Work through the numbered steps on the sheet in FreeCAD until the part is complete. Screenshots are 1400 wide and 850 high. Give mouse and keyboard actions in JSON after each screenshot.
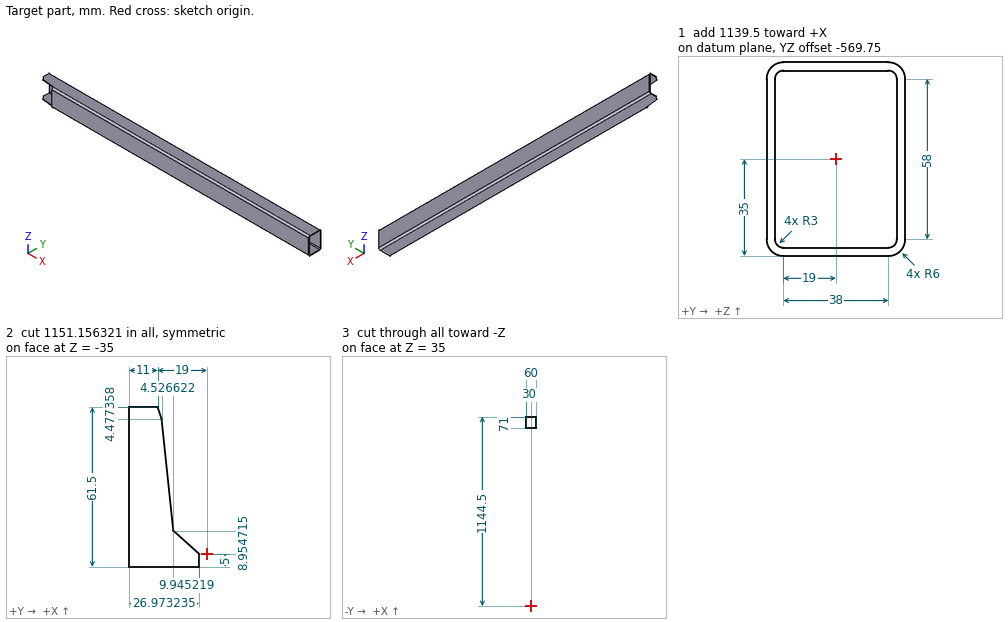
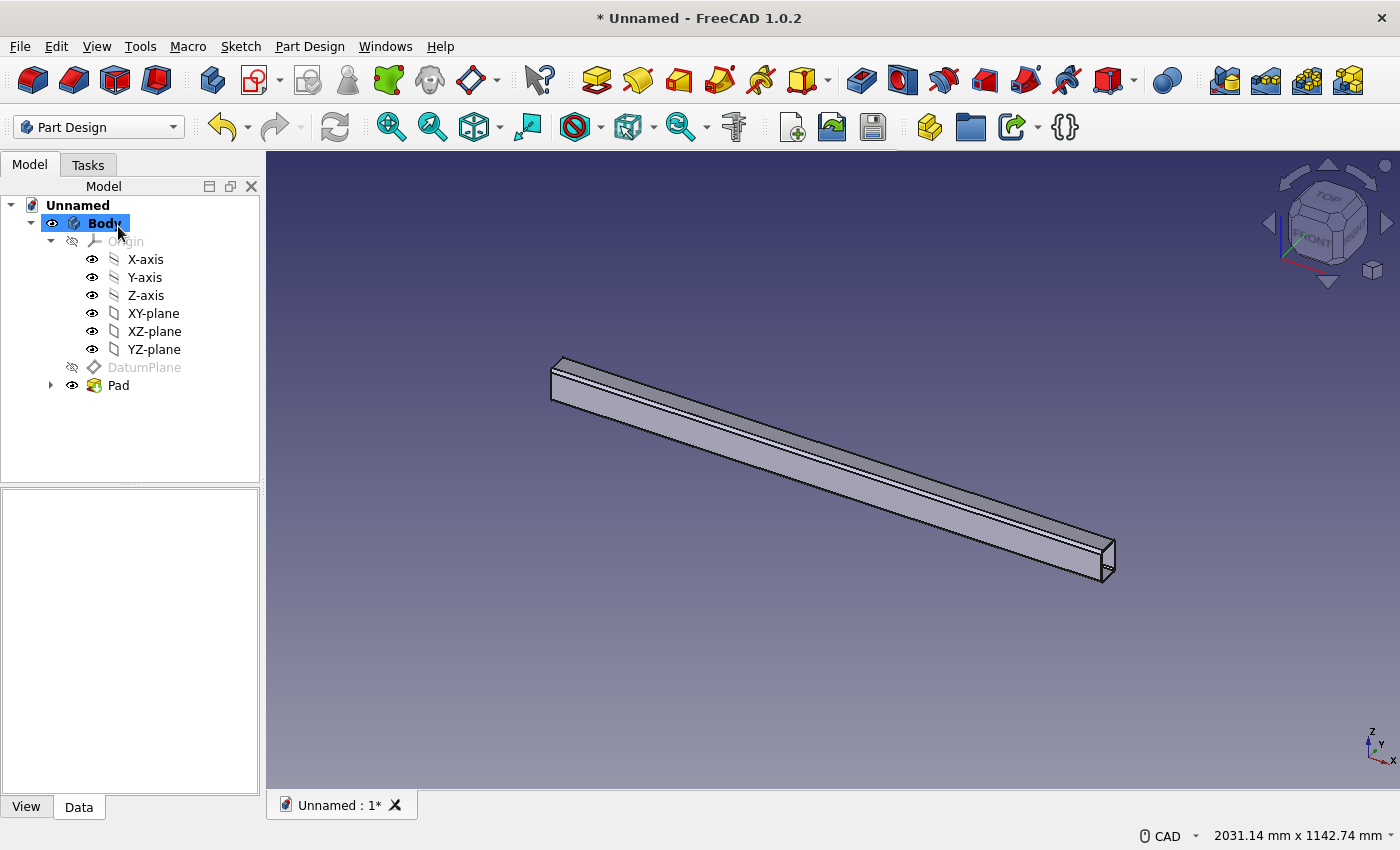
{"action": "key", "text": "5"}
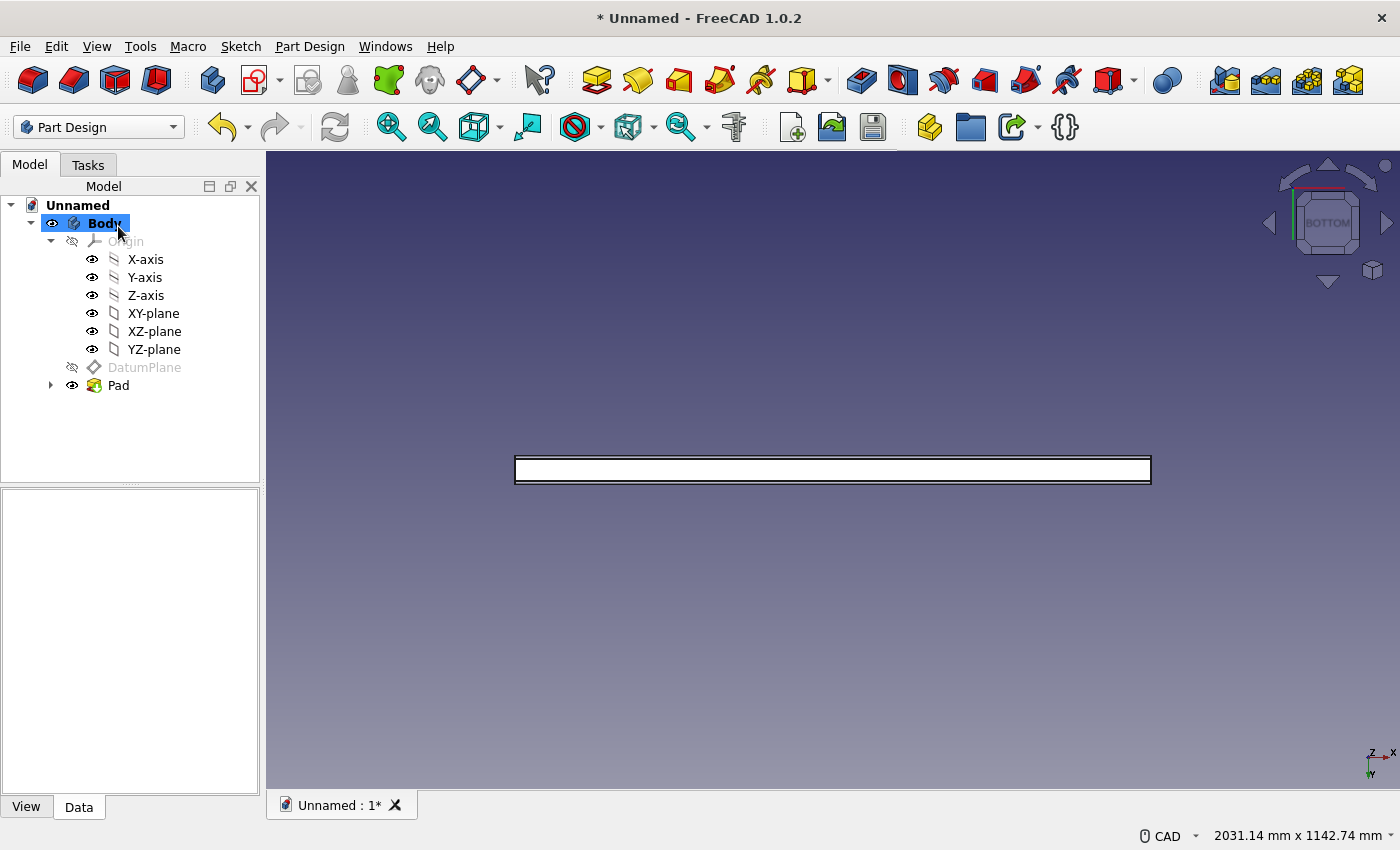
{"action": "left_click", "coordinate": [833, 469]}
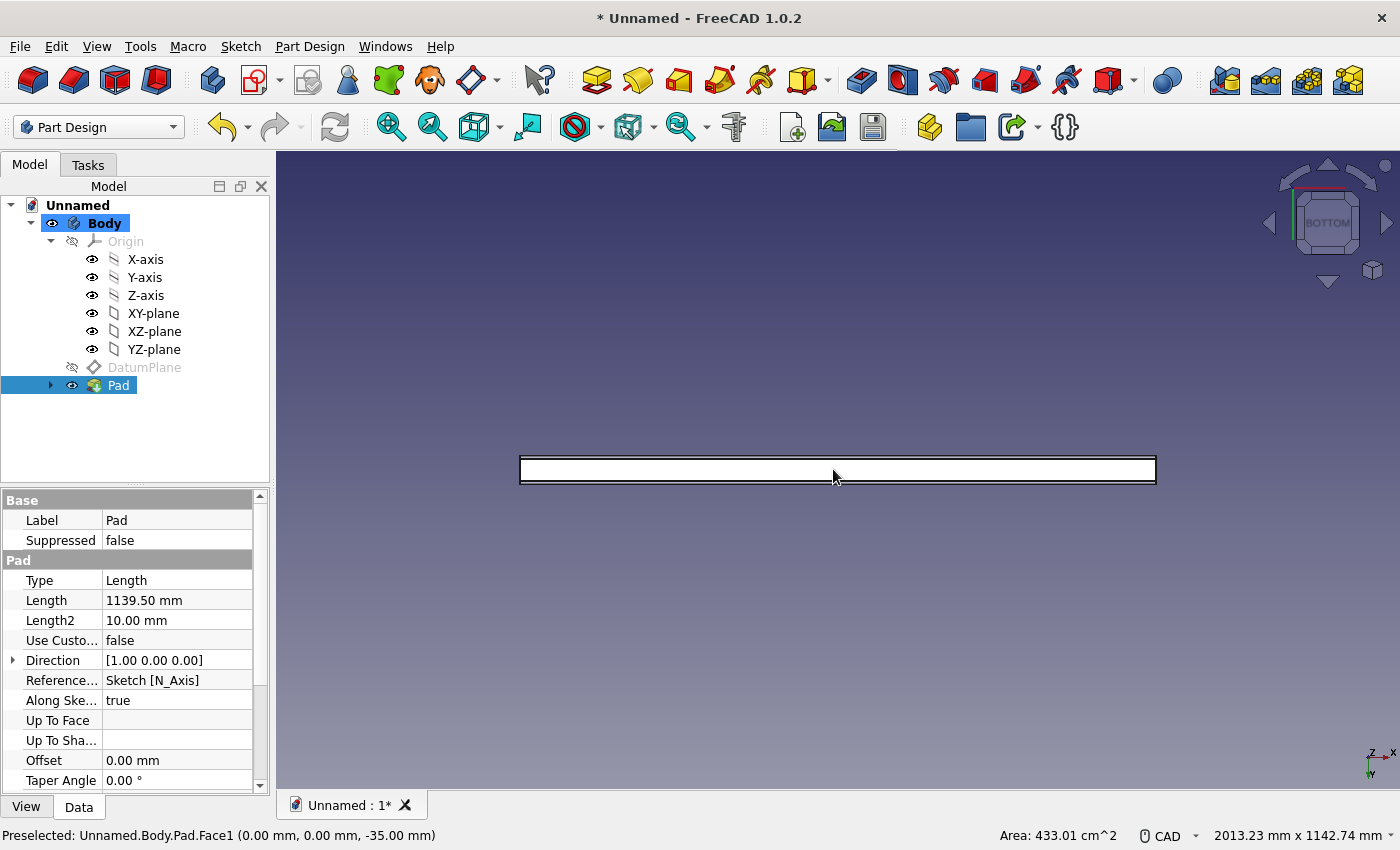
{"action": "left_click", "coordinate": [254, 80]}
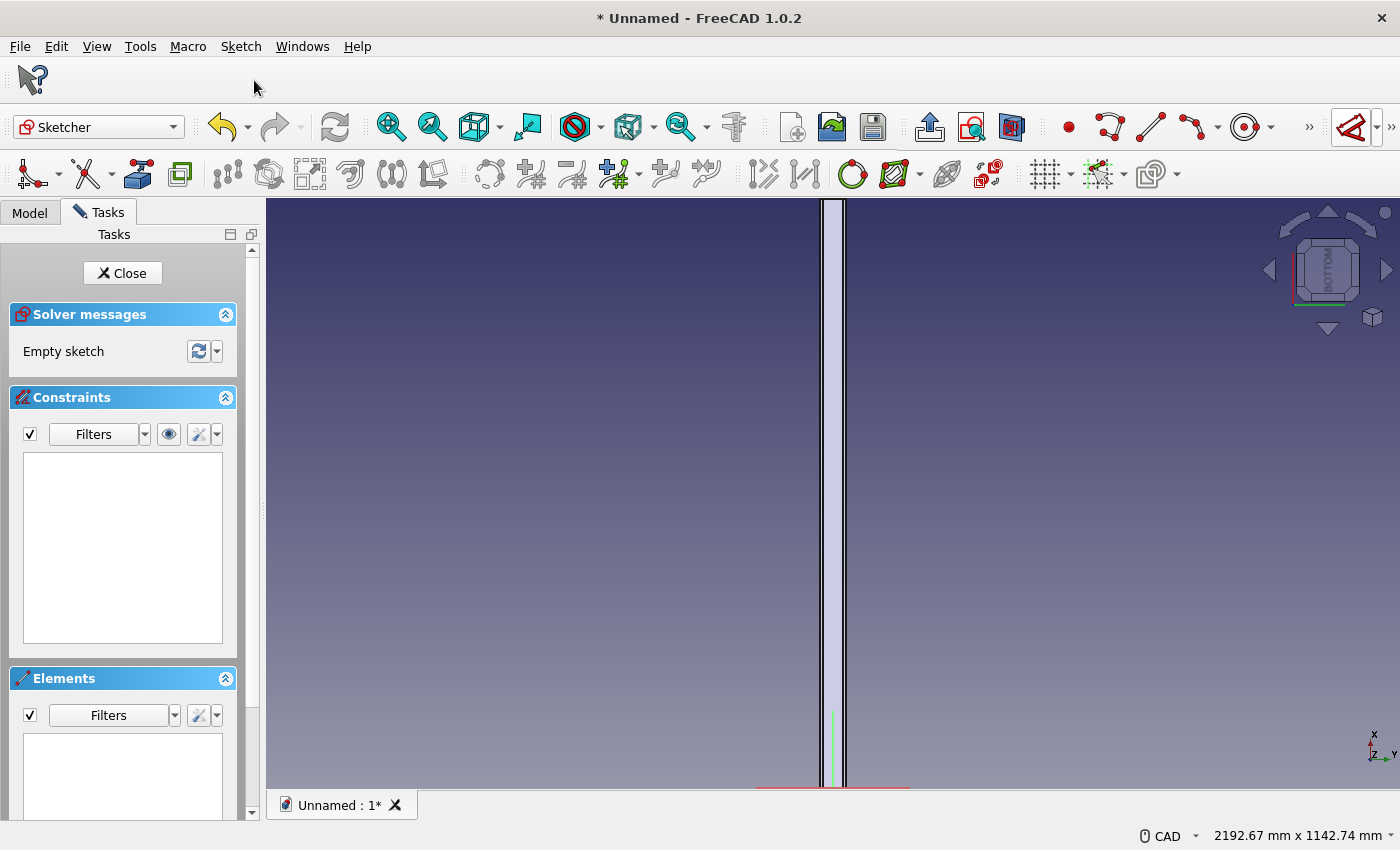
{"action": "scroll", "coordinate": [764, 494], "scroll_direction": "down", "scroll_amount": 5}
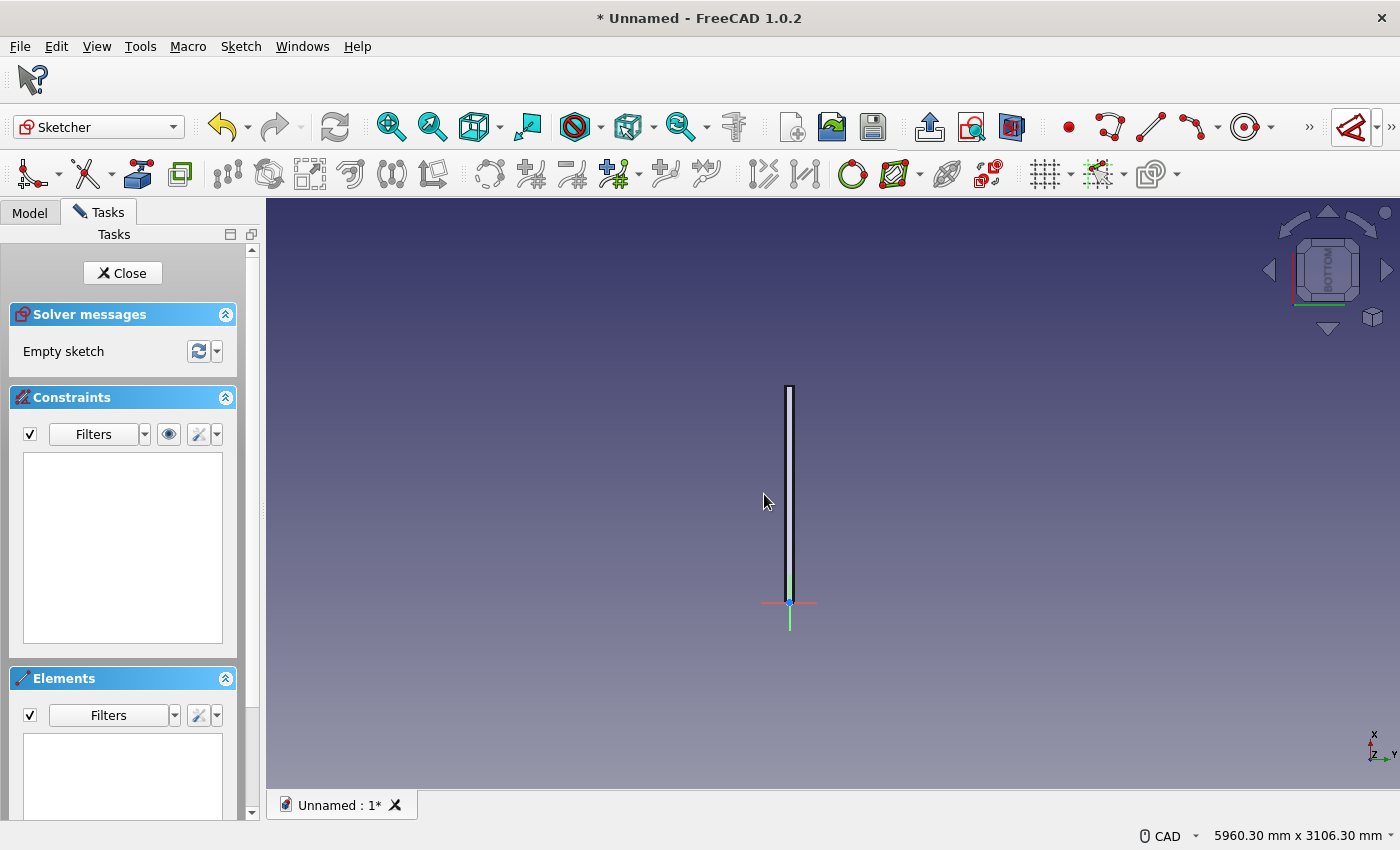
{"action": "scroll", "coordinate": [788, 603], "scroll_direction": "up", "scroll_amount": 15}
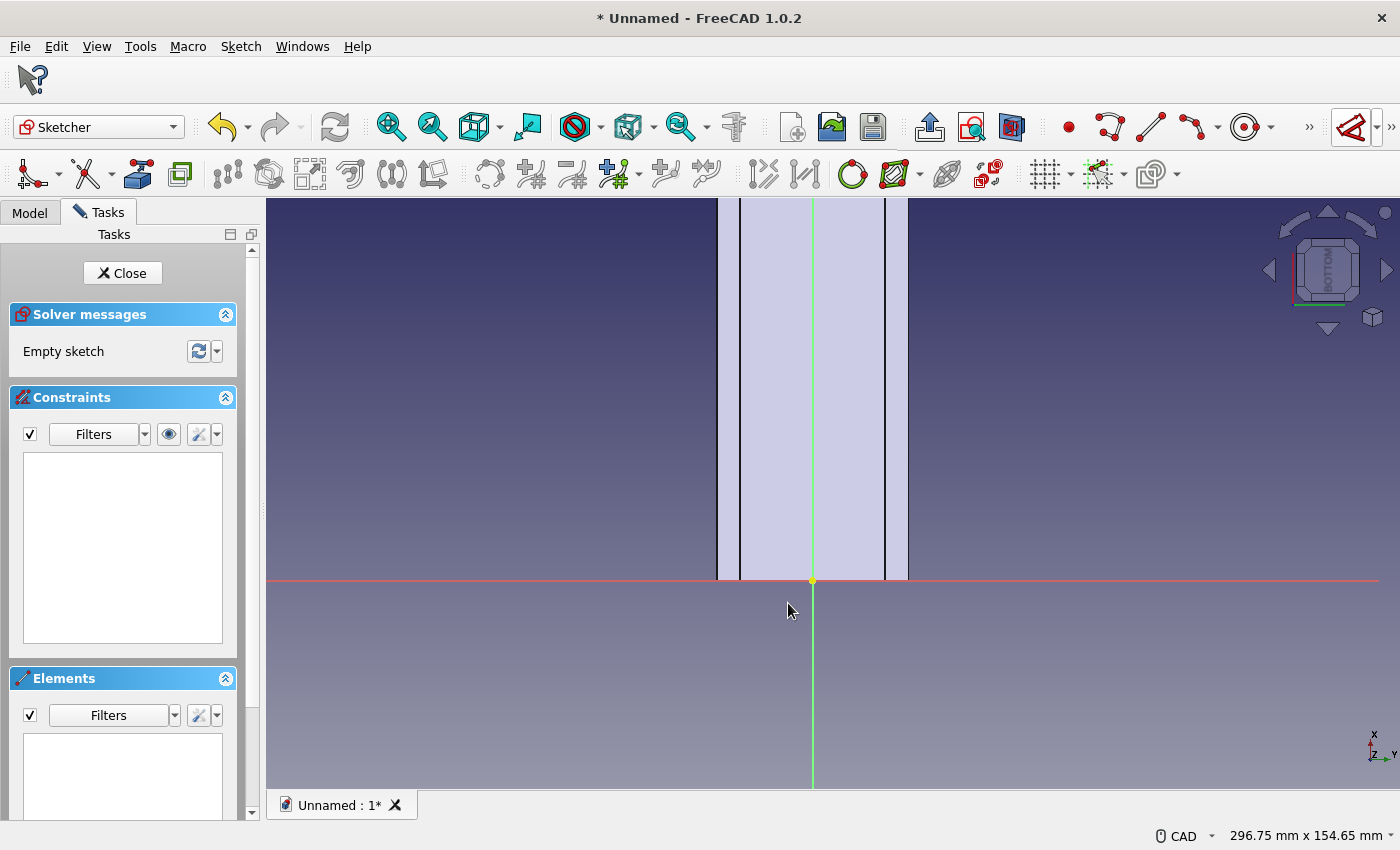
{"action": "scroll", "coordinate": [736, 459], "scroll_direction": "up", "scroll_amount": 2}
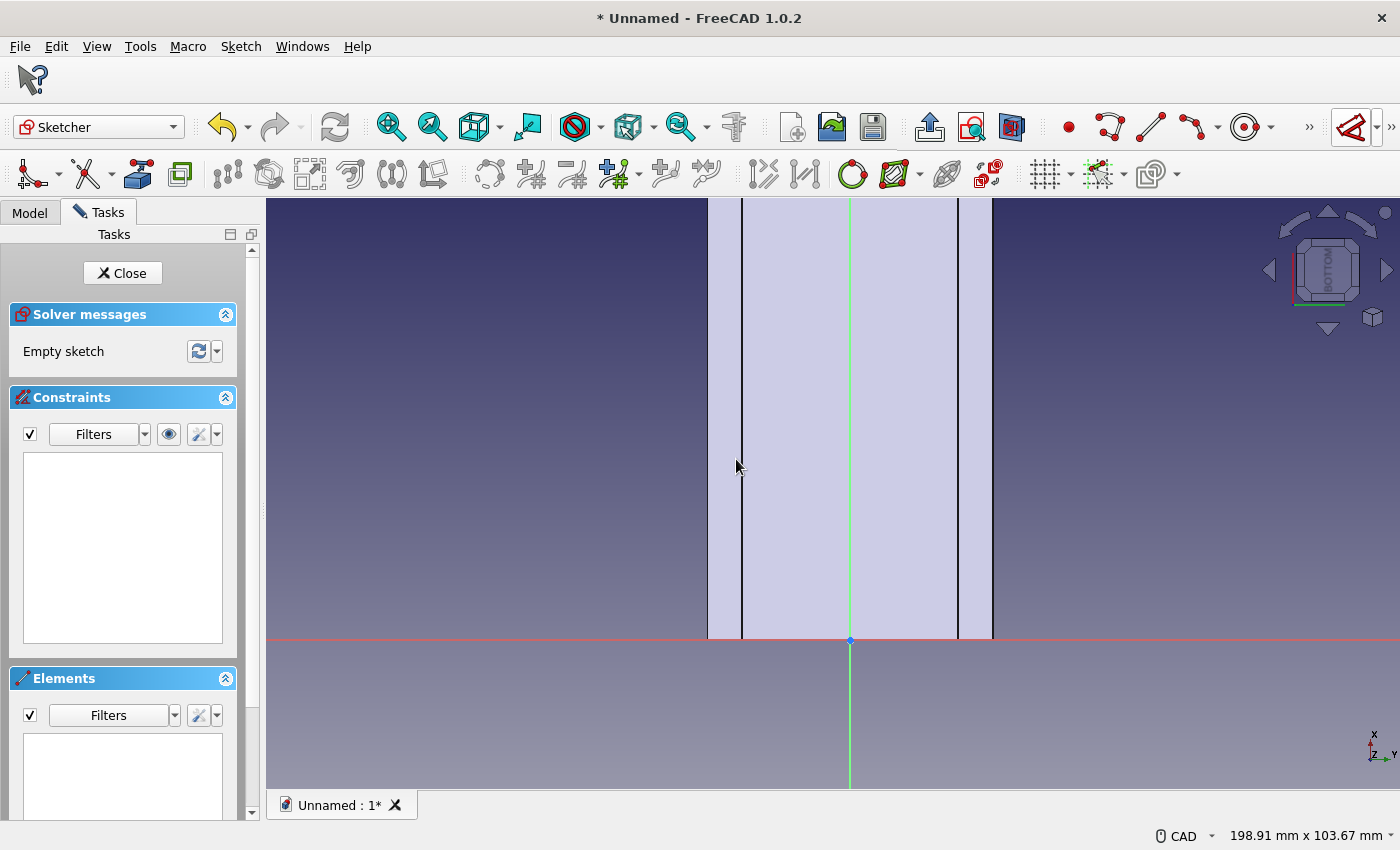
{"action": "key", "text": "g m"}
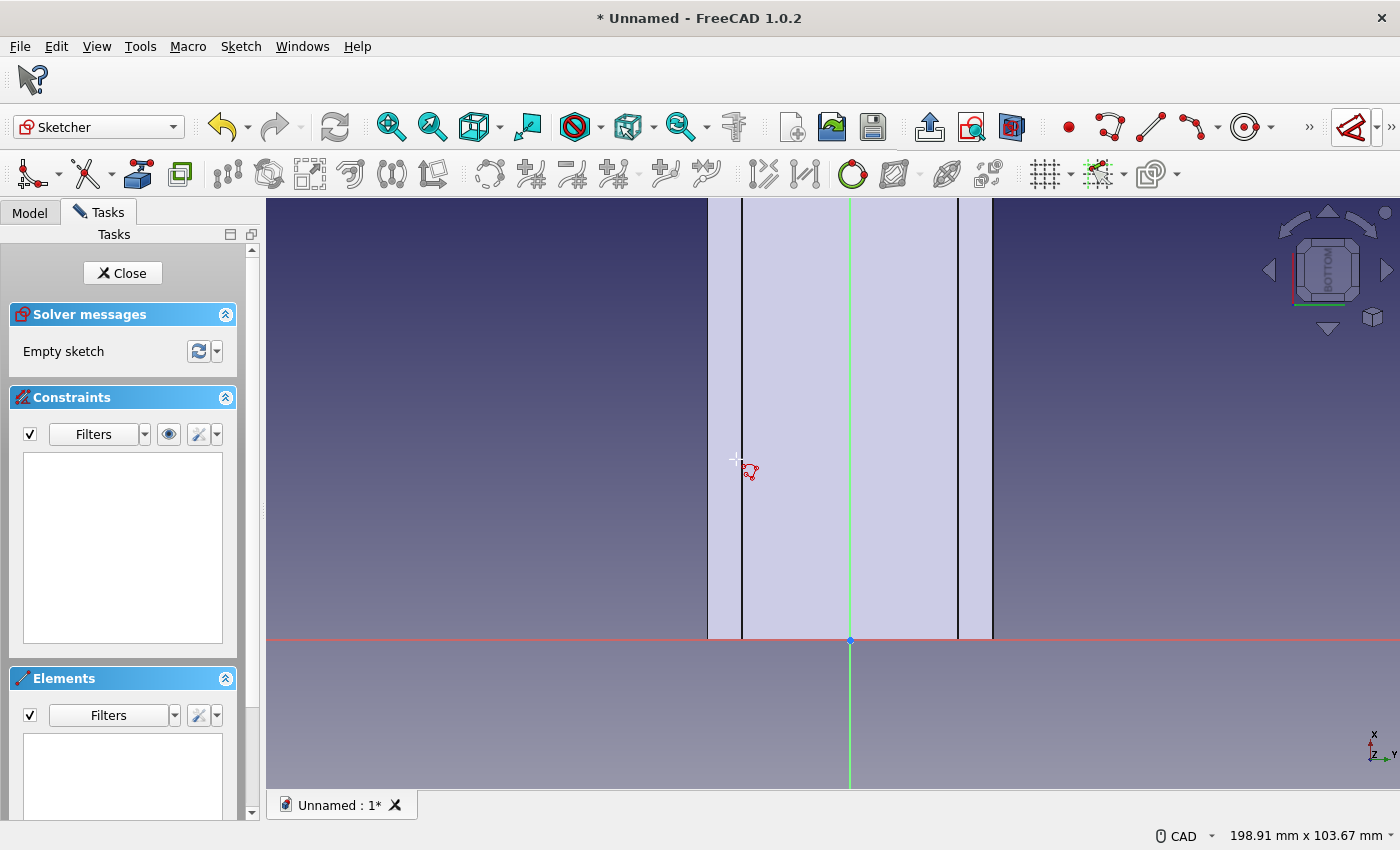
{"action": "left_click", "coordinate": [833, 640]}
{"action": "left_click", "coordinate": [776, 589]}
{"action": "left_click", "coordinate": [750, 343]}
{"action": "left_click", "coordinate": [742, 318]}
{"action": "left_click", "coordinate": [679, 318]}
{"action": "left_click", "coordinate": [679, 669]}
{"action": "left_click", "coordinate": [833, 669]}
{"action": "left_click", "coordinate": [833, 640]}
{"action": "key", "text": "Escape"}
{"action": "key", "text": "Escape"}